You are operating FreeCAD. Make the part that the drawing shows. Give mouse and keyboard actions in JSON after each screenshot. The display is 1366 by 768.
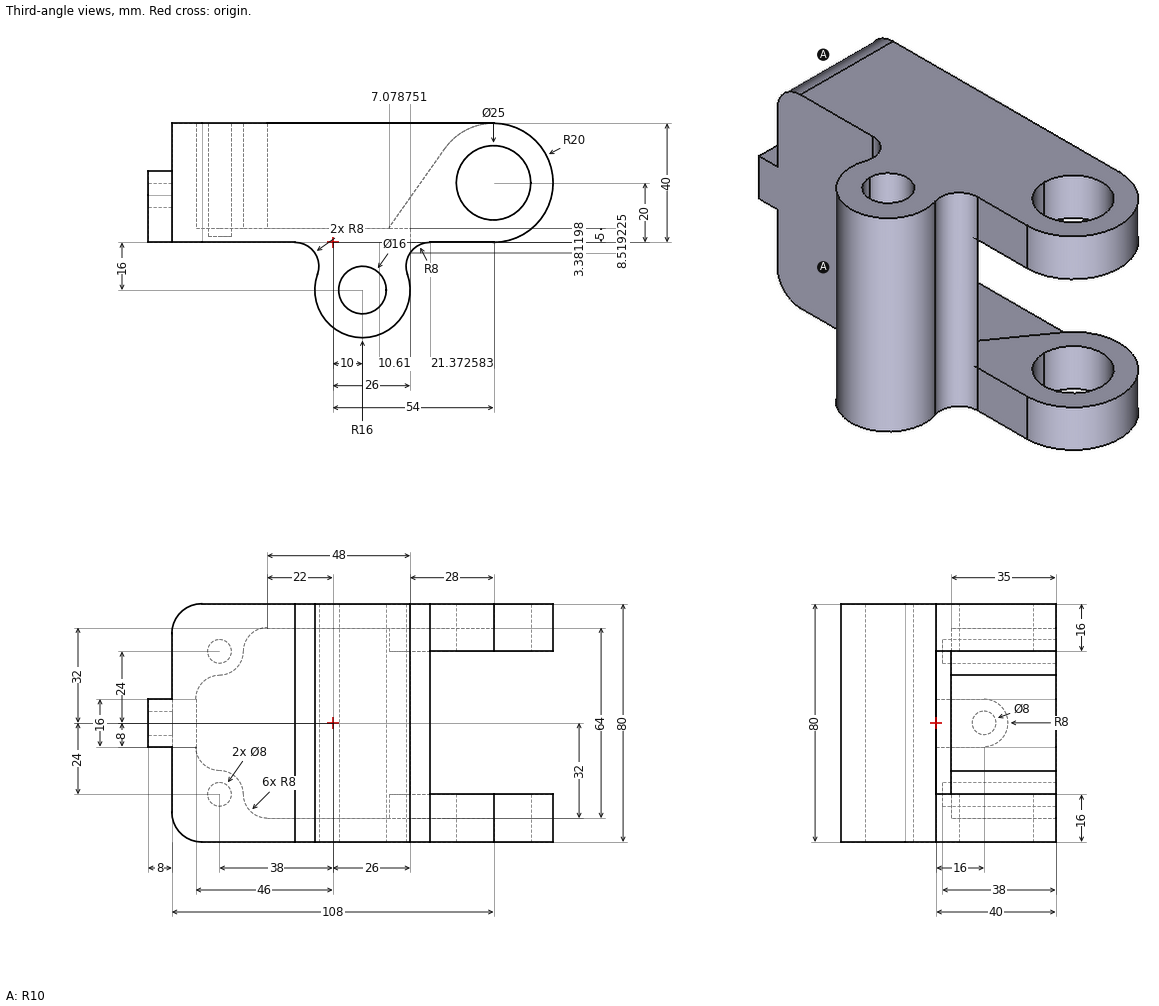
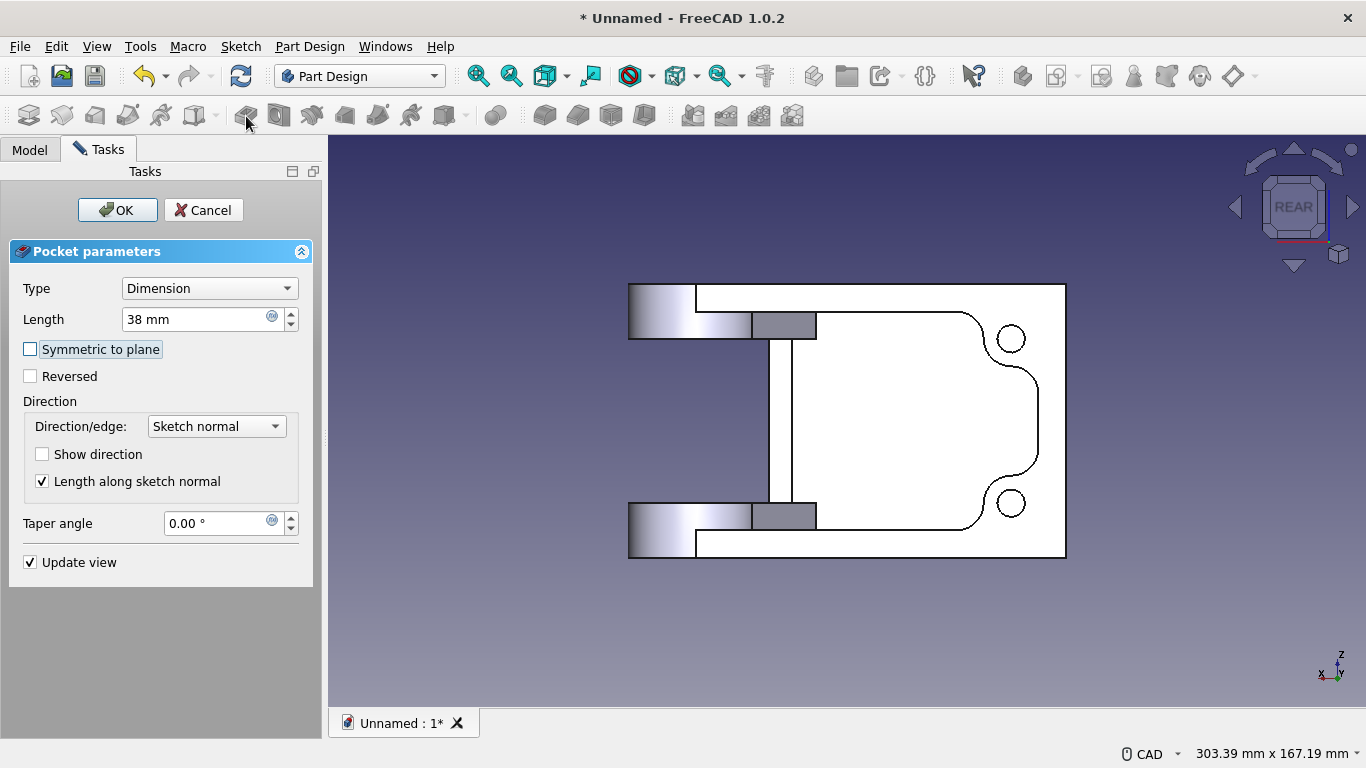
{"action": "left_click", "coordinate": [118, 210]}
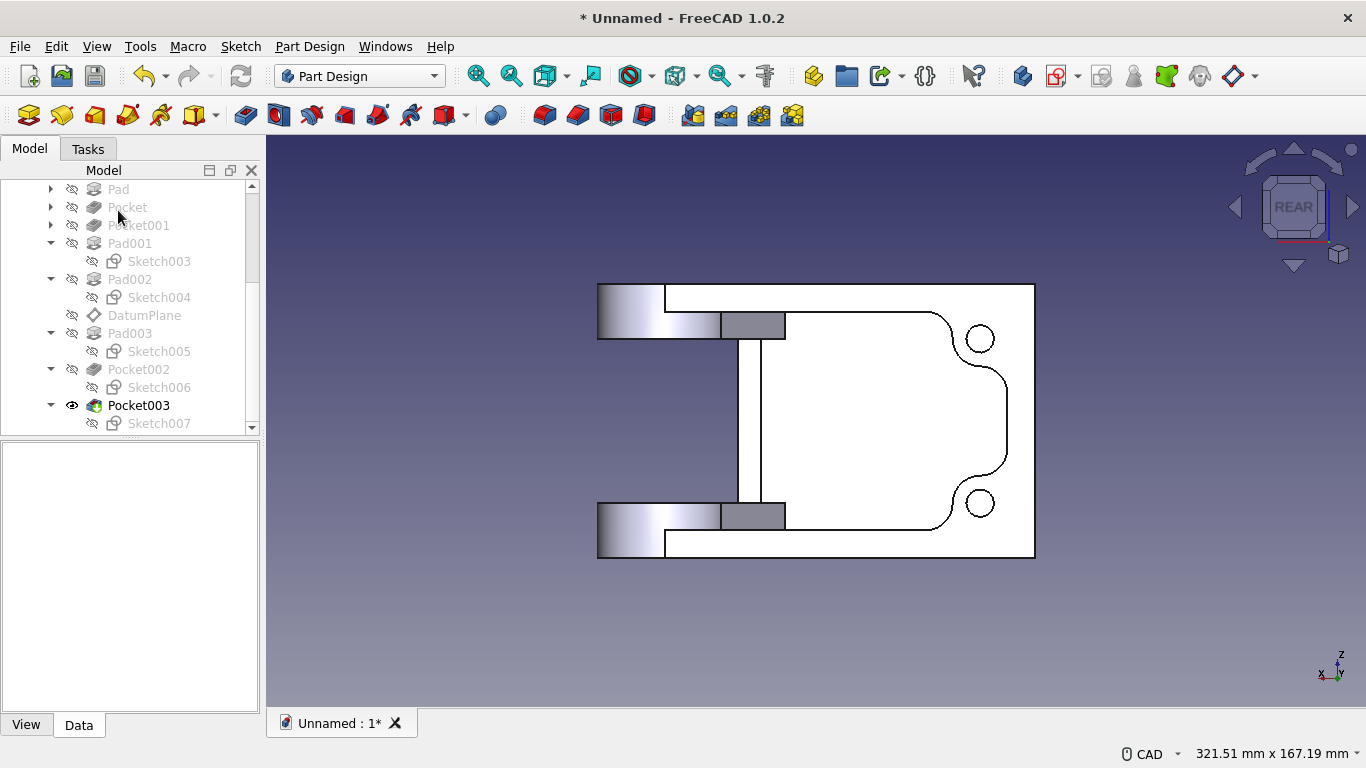
{"action": "key", "text": "0"}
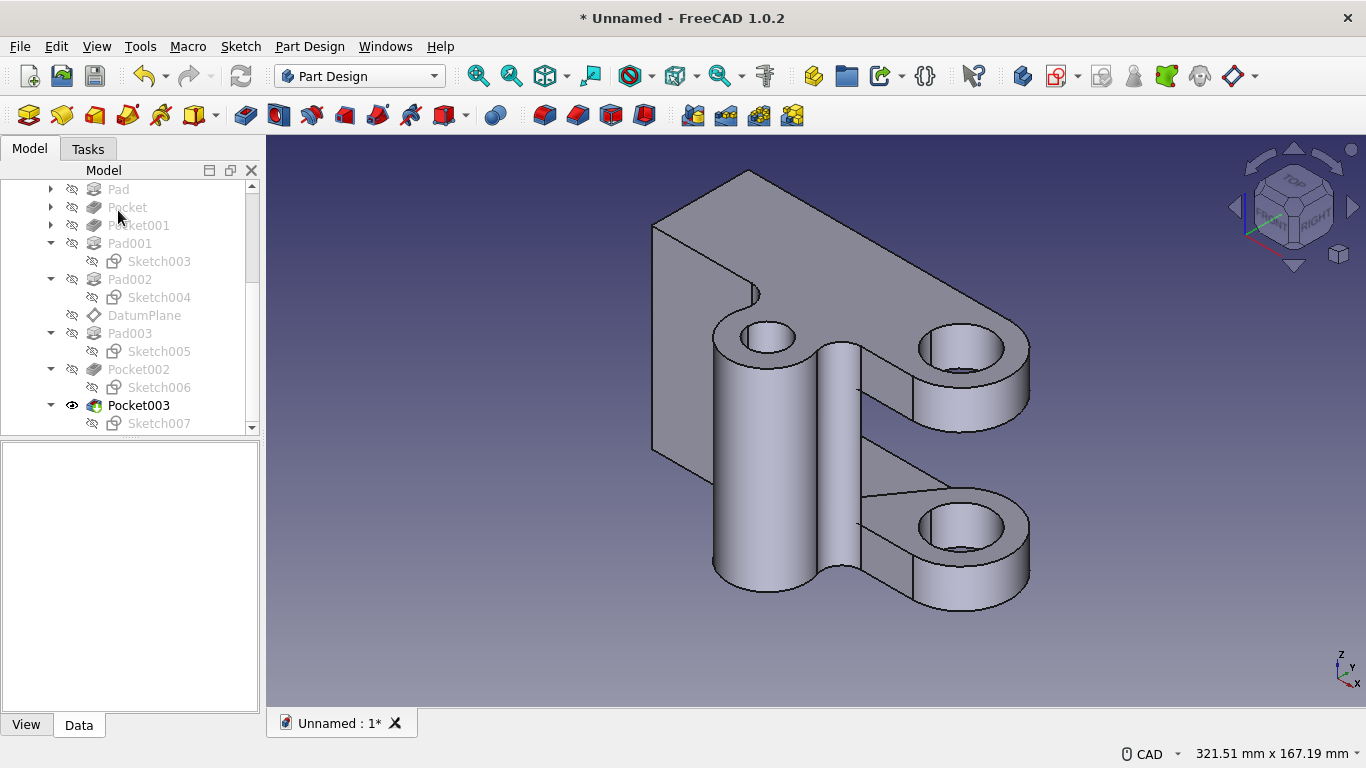
{"action": "key", "text": "2"}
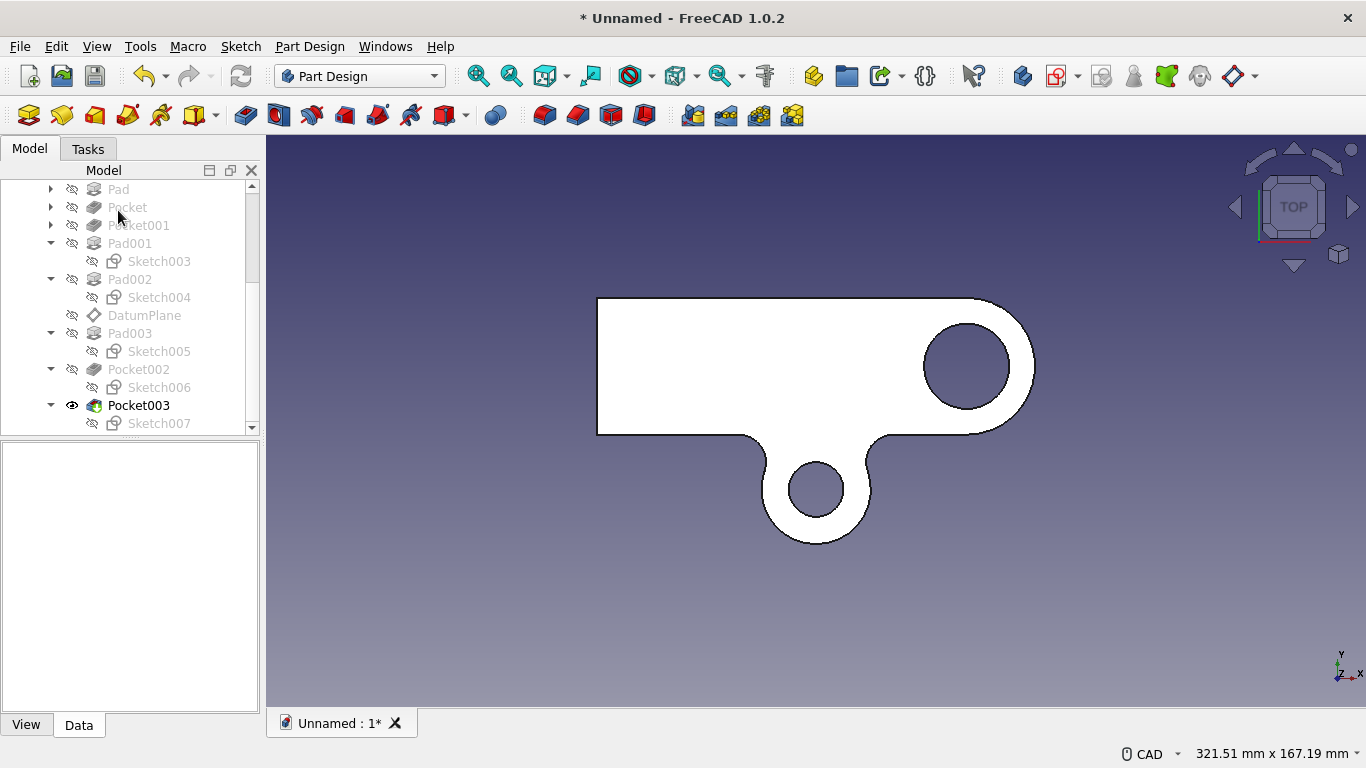
{"action": "key", "text": "v f"}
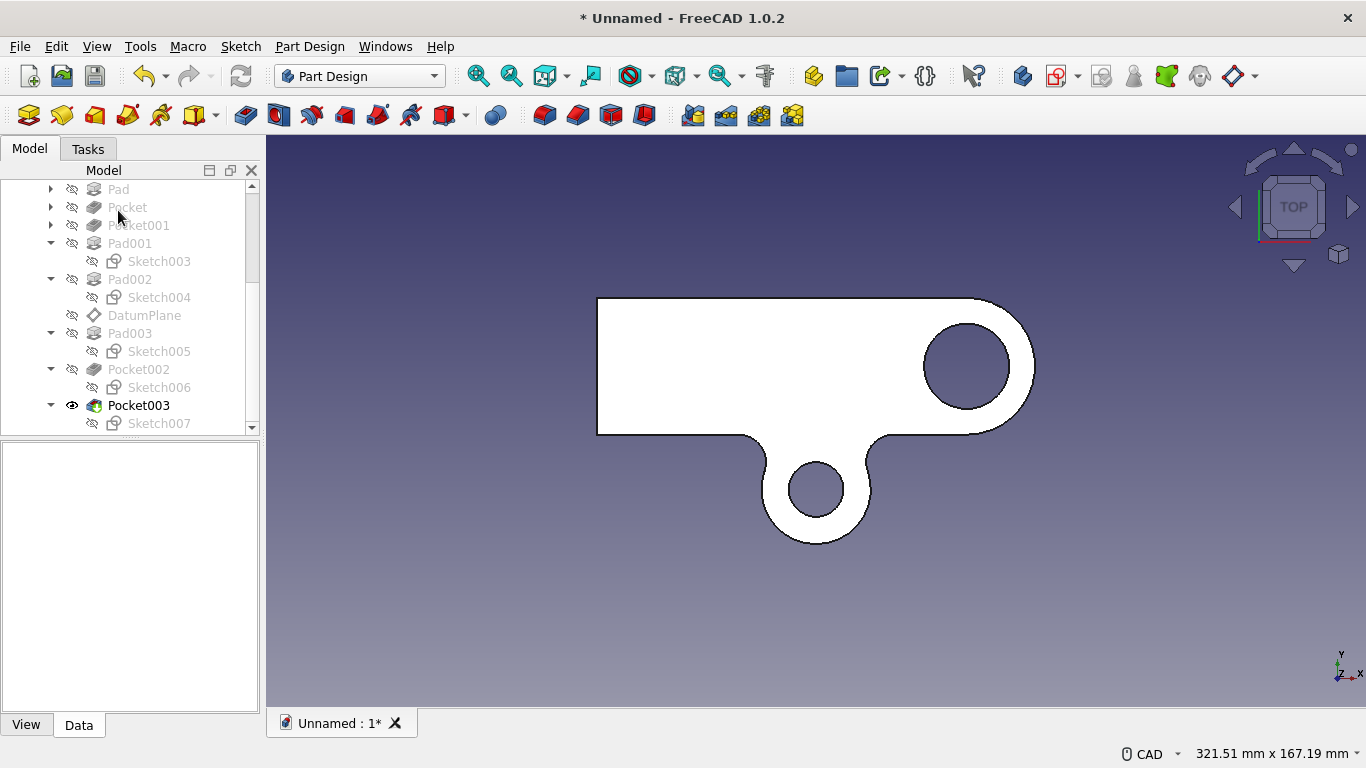
{"action": "left_click", "coordinate": [597, 365]}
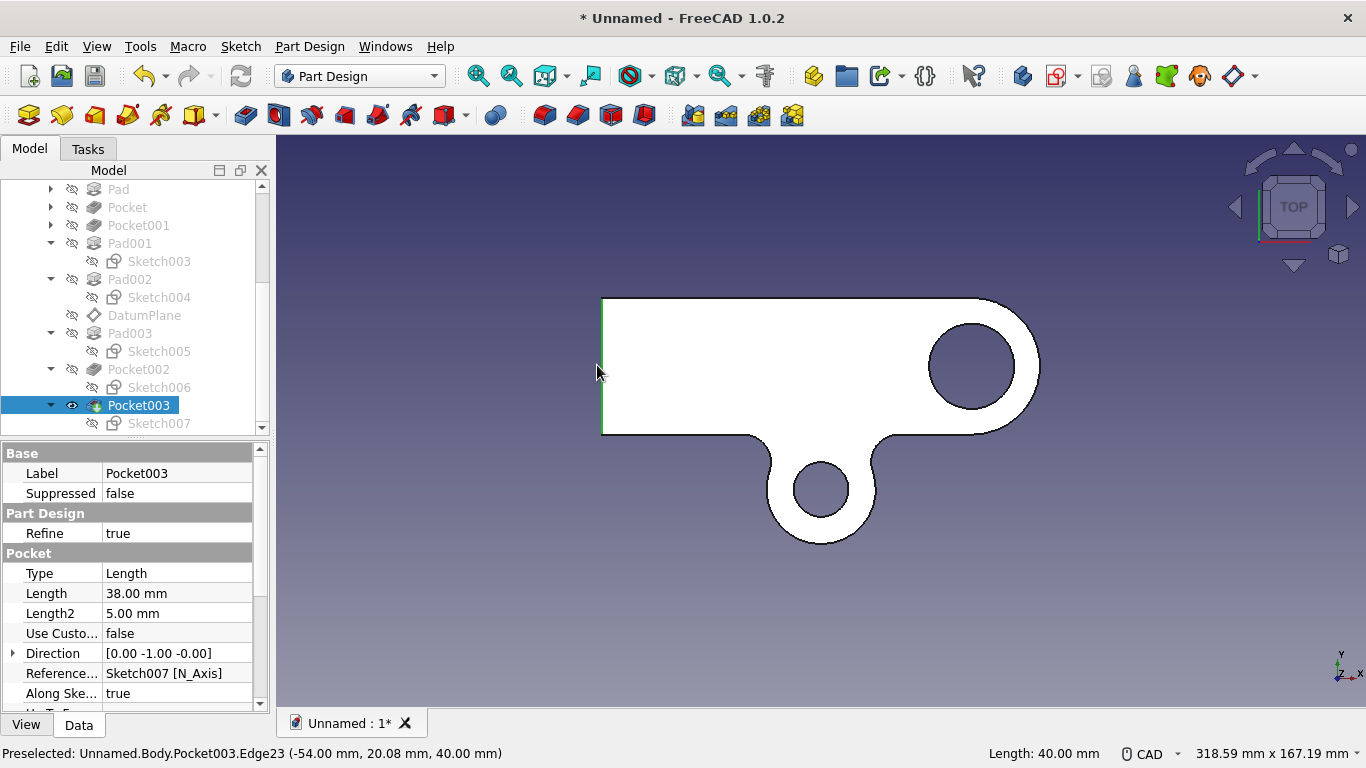
{"action": "key", "text": "1"}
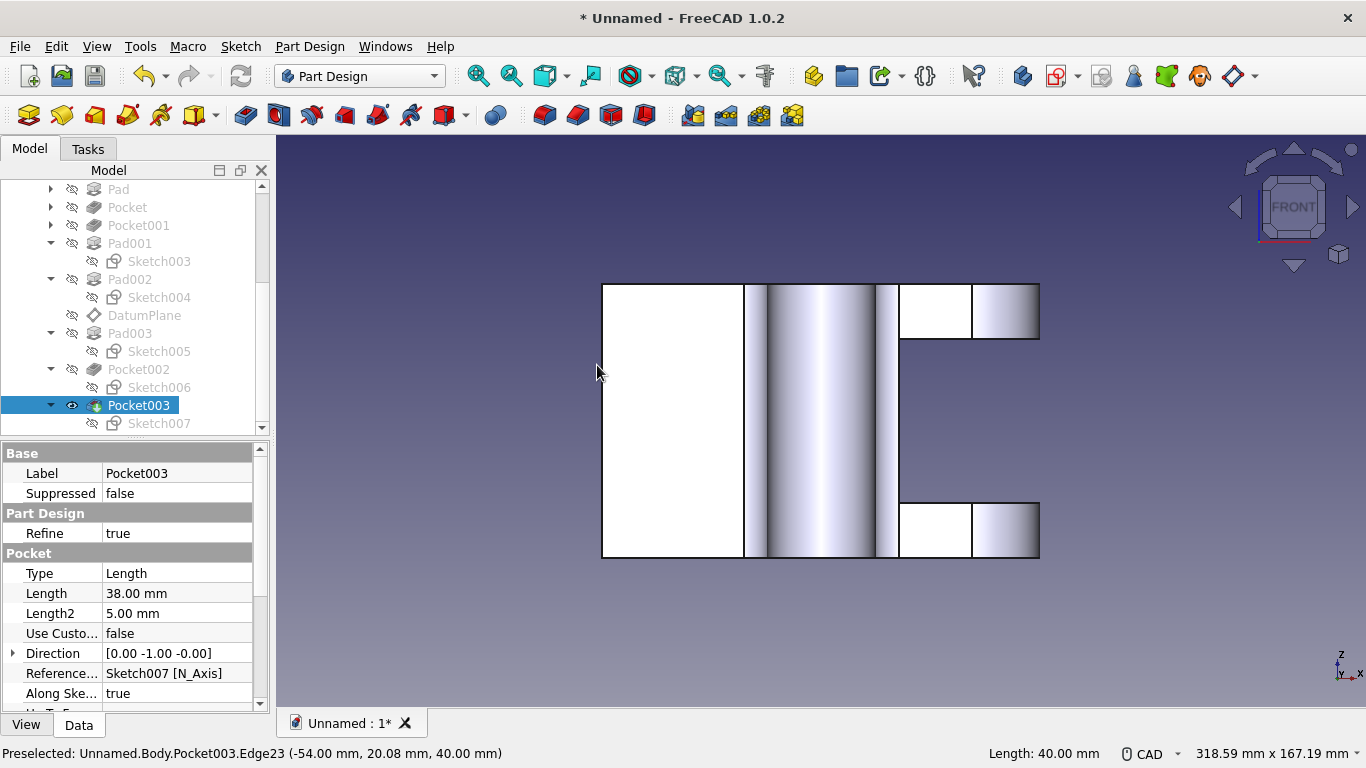
{"action": "key", "text": "3"}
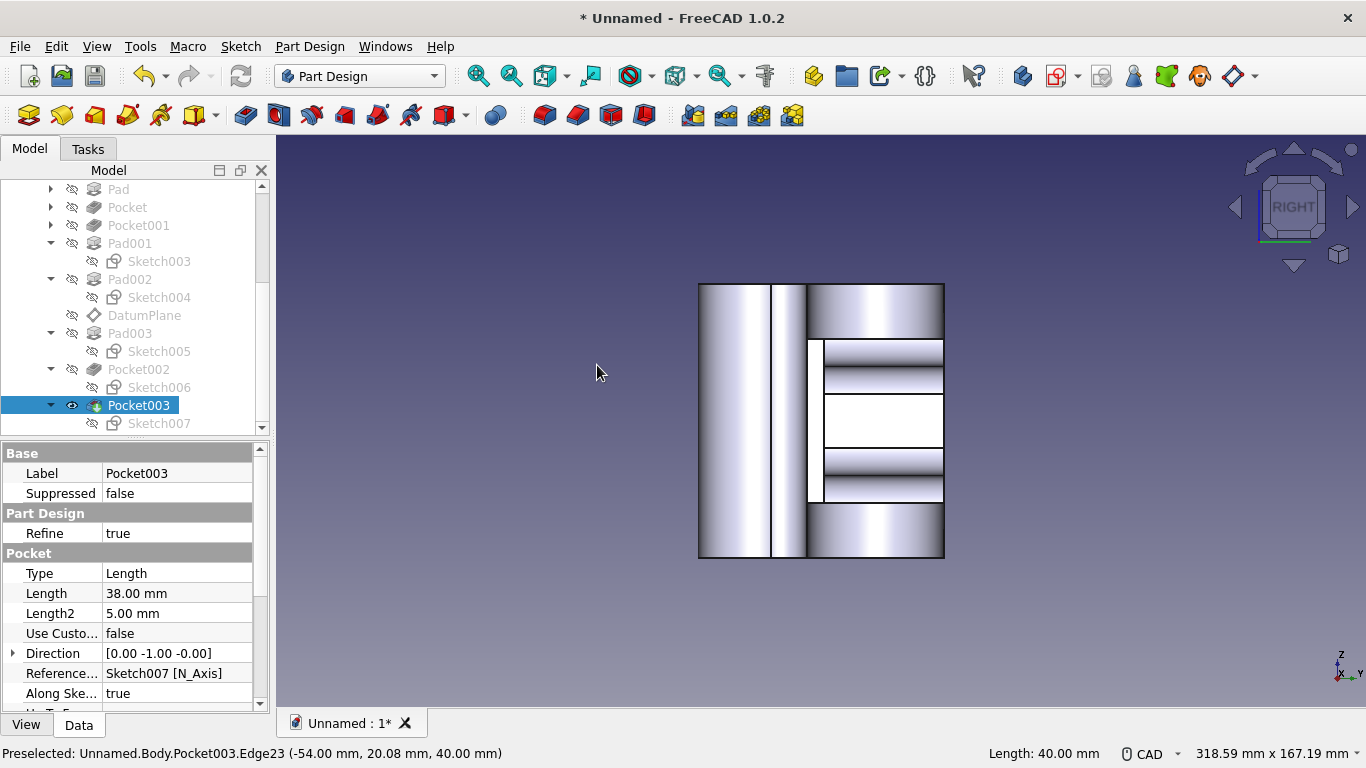
{"action": "key", "text": "5"}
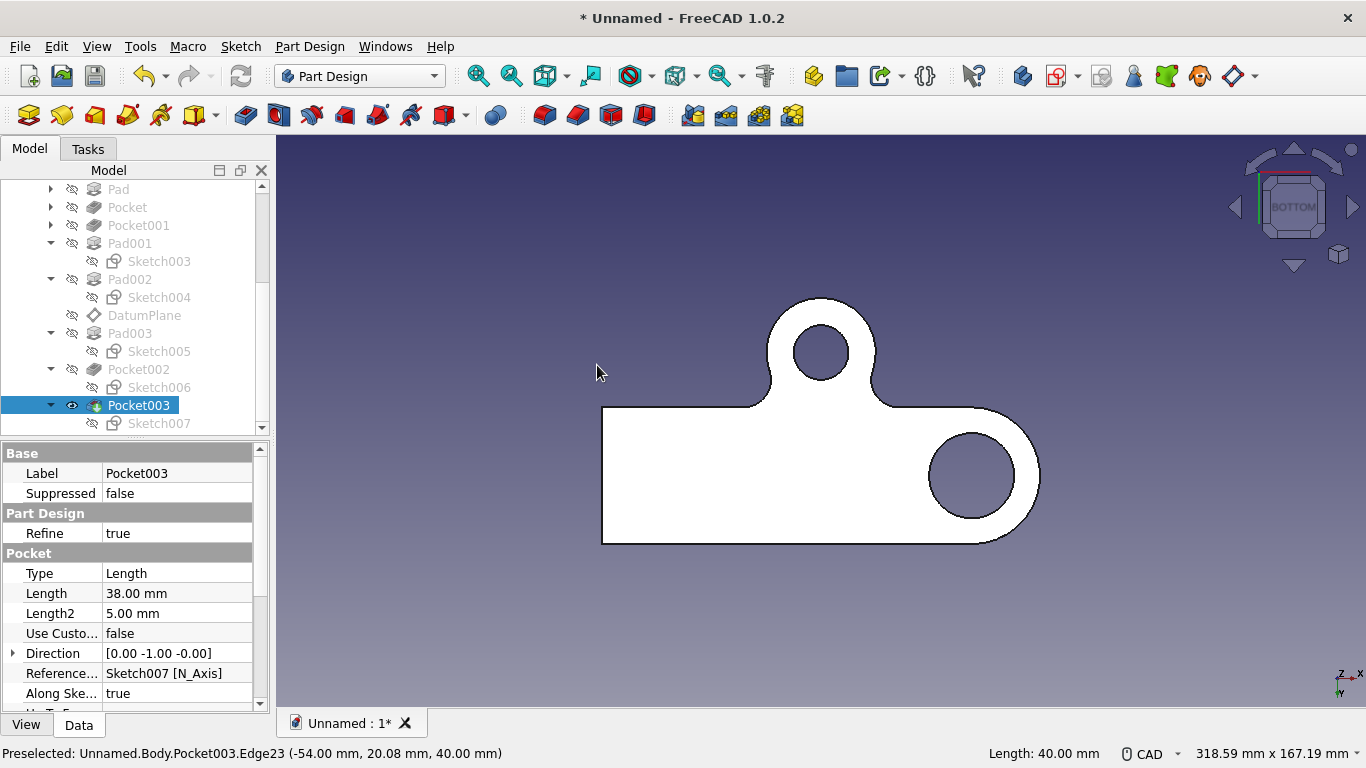
{"action": "key", "text": "v f"}